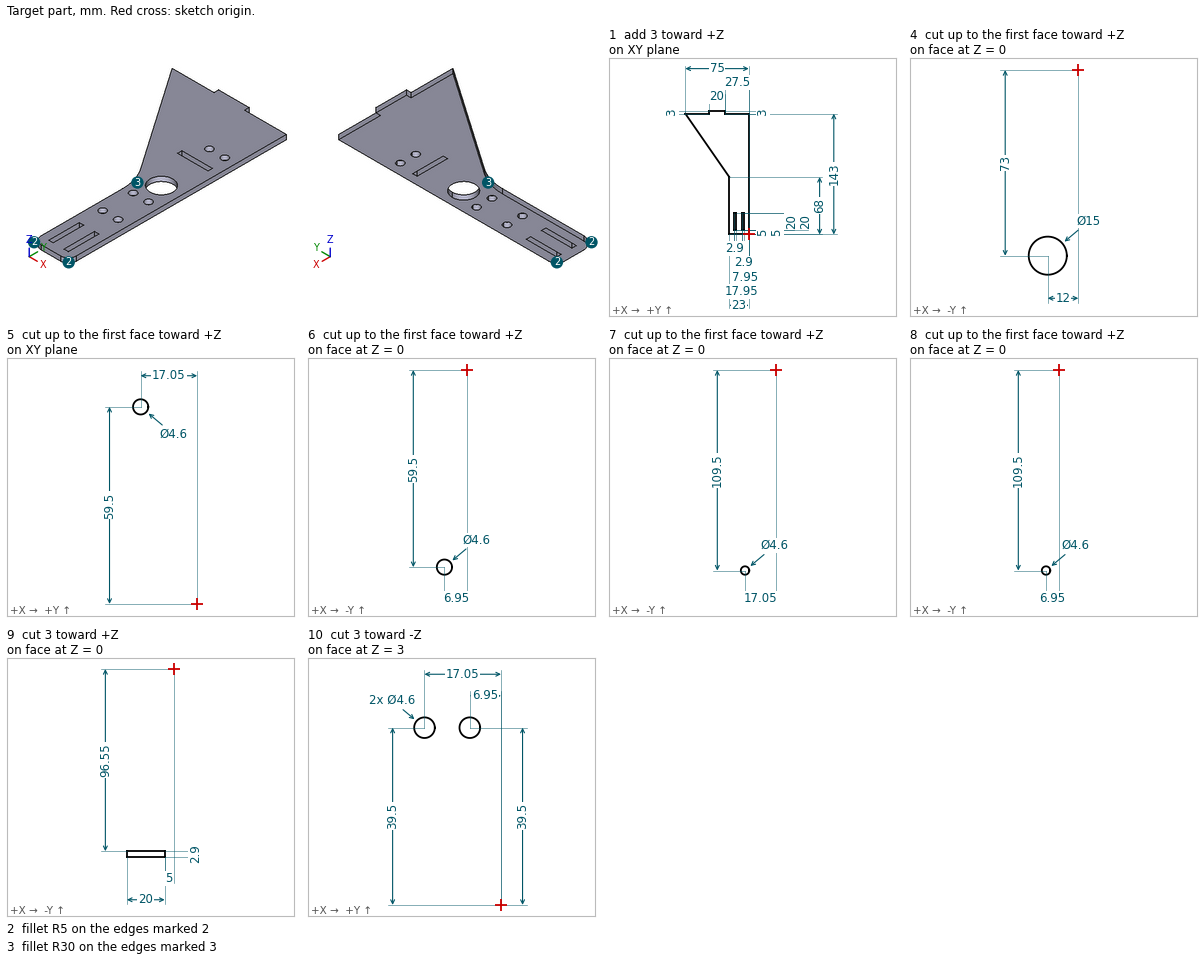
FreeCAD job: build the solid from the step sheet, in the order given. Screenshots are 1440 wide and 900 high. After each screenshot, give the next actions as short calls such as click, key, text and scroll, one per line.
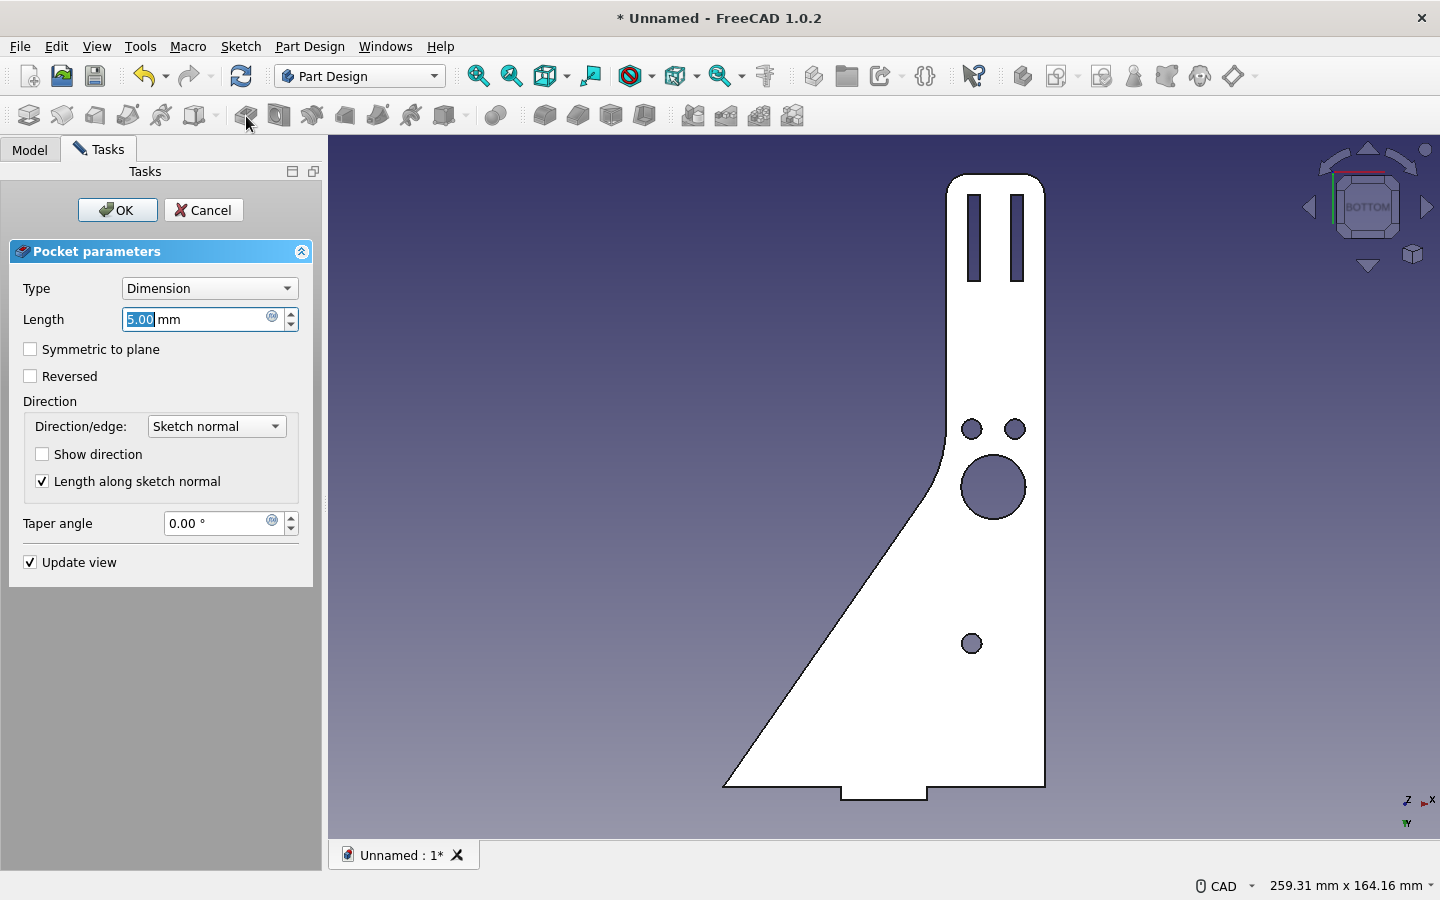
click(210, 288)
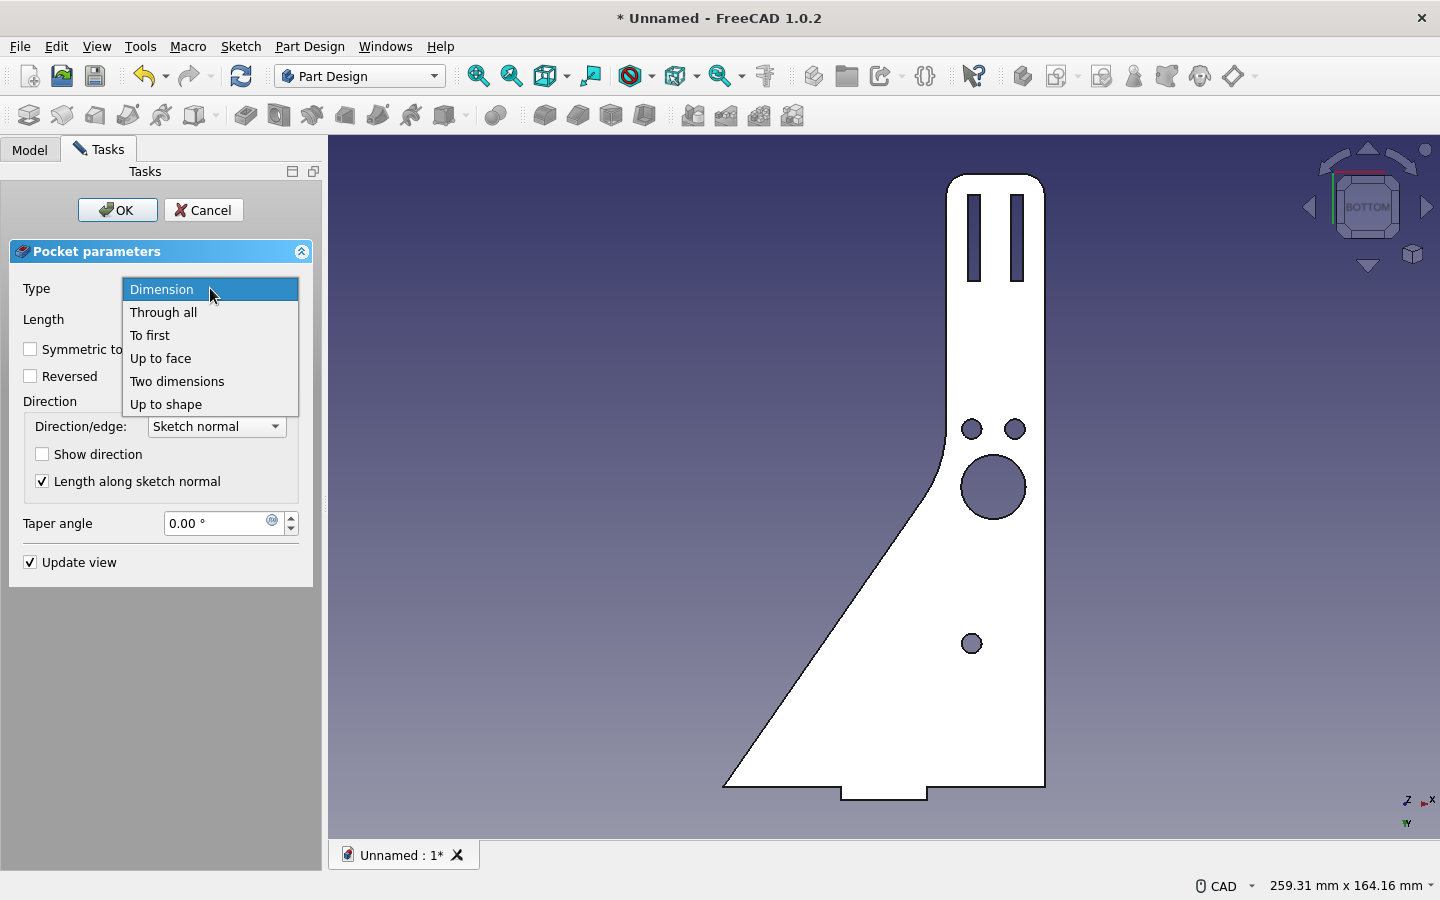
click(208, 336)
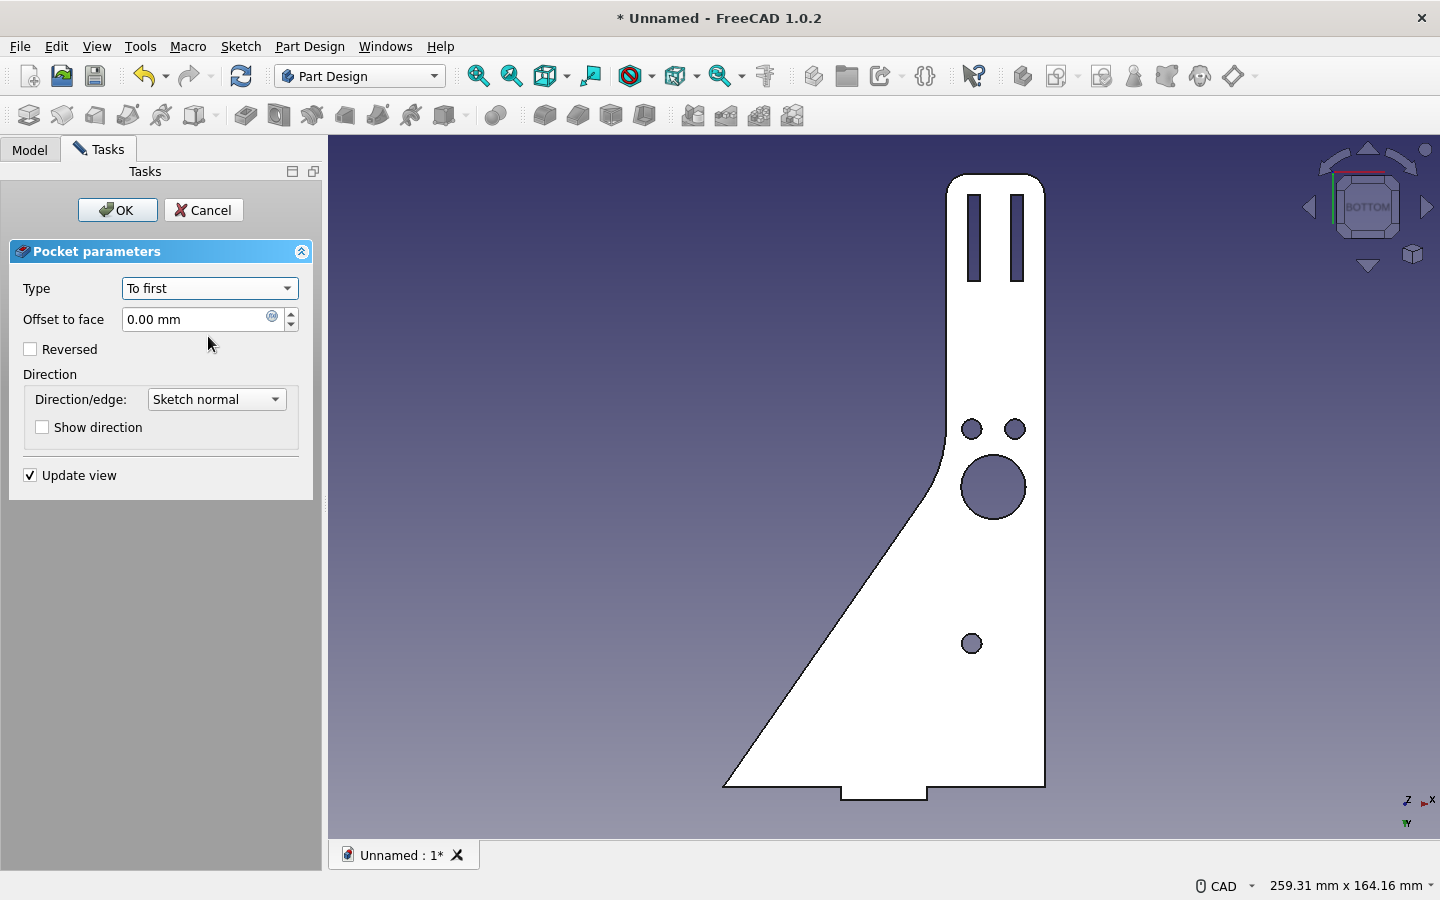
click(118, 210)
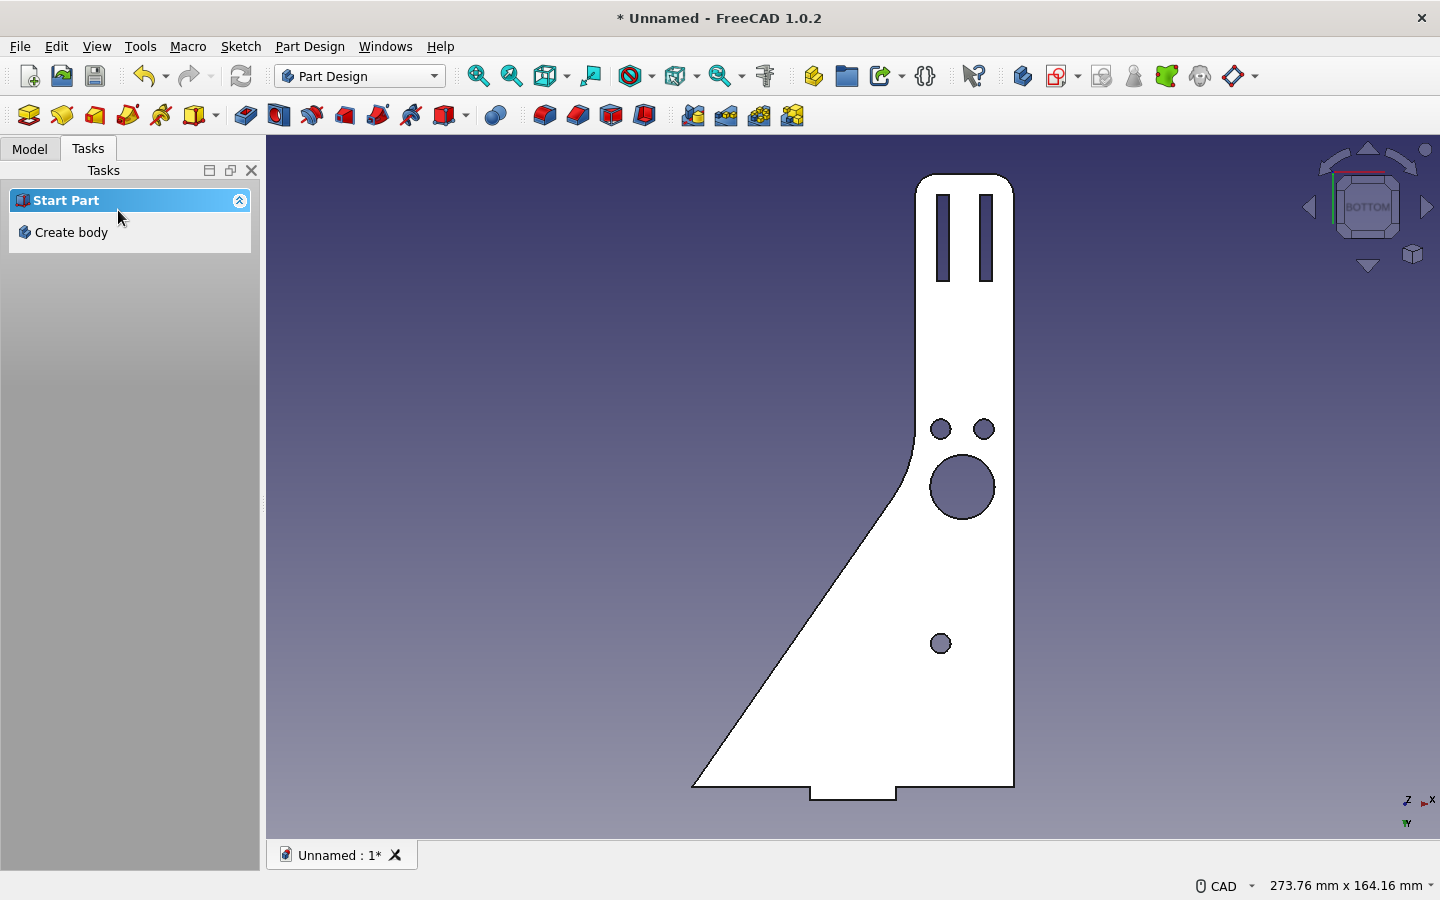
click(853, 665)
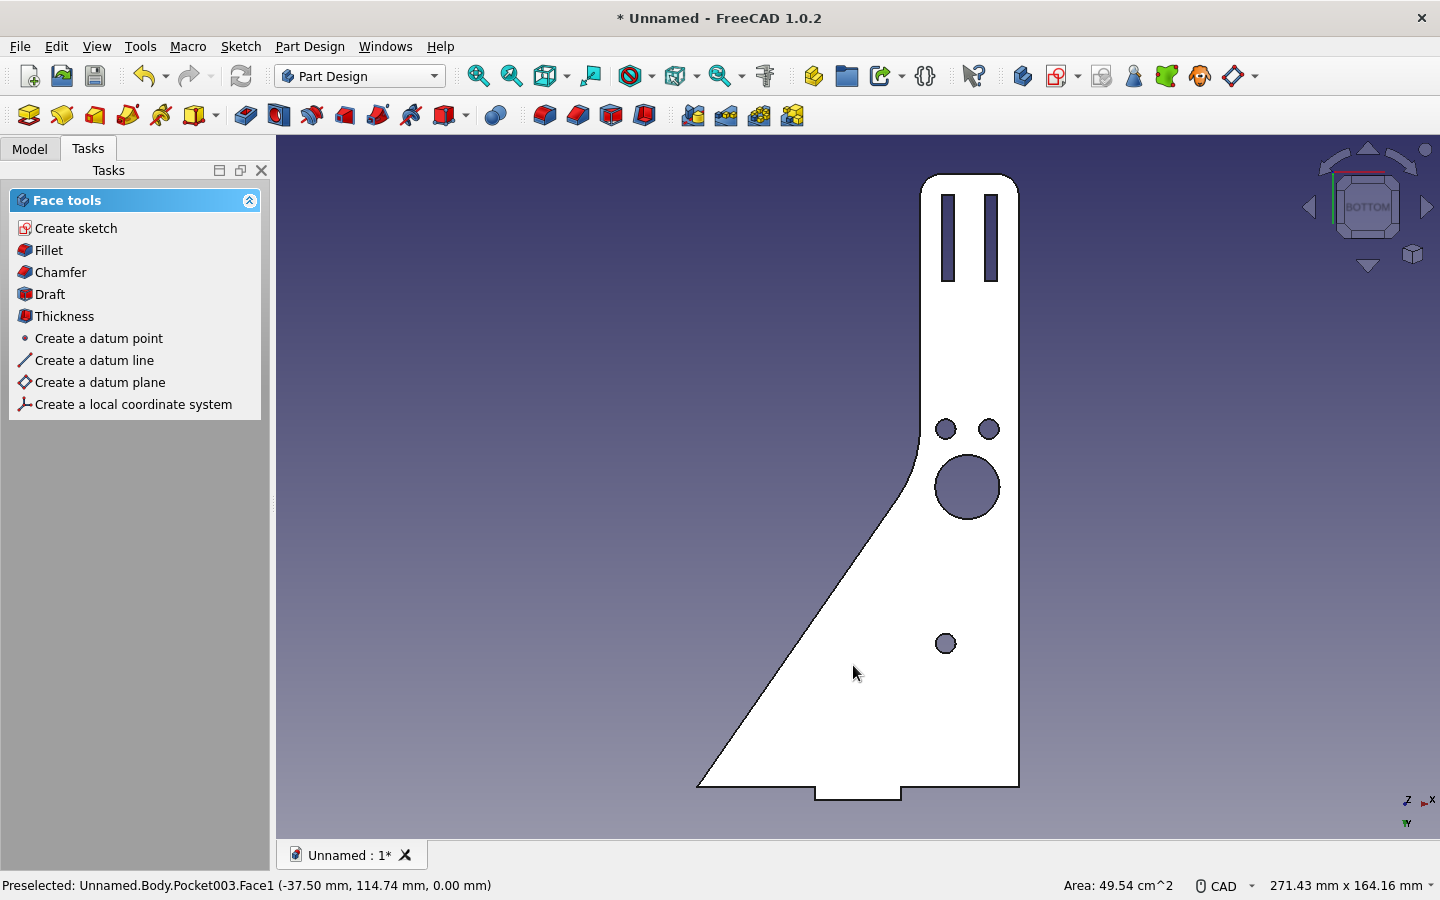
click(1056, 76)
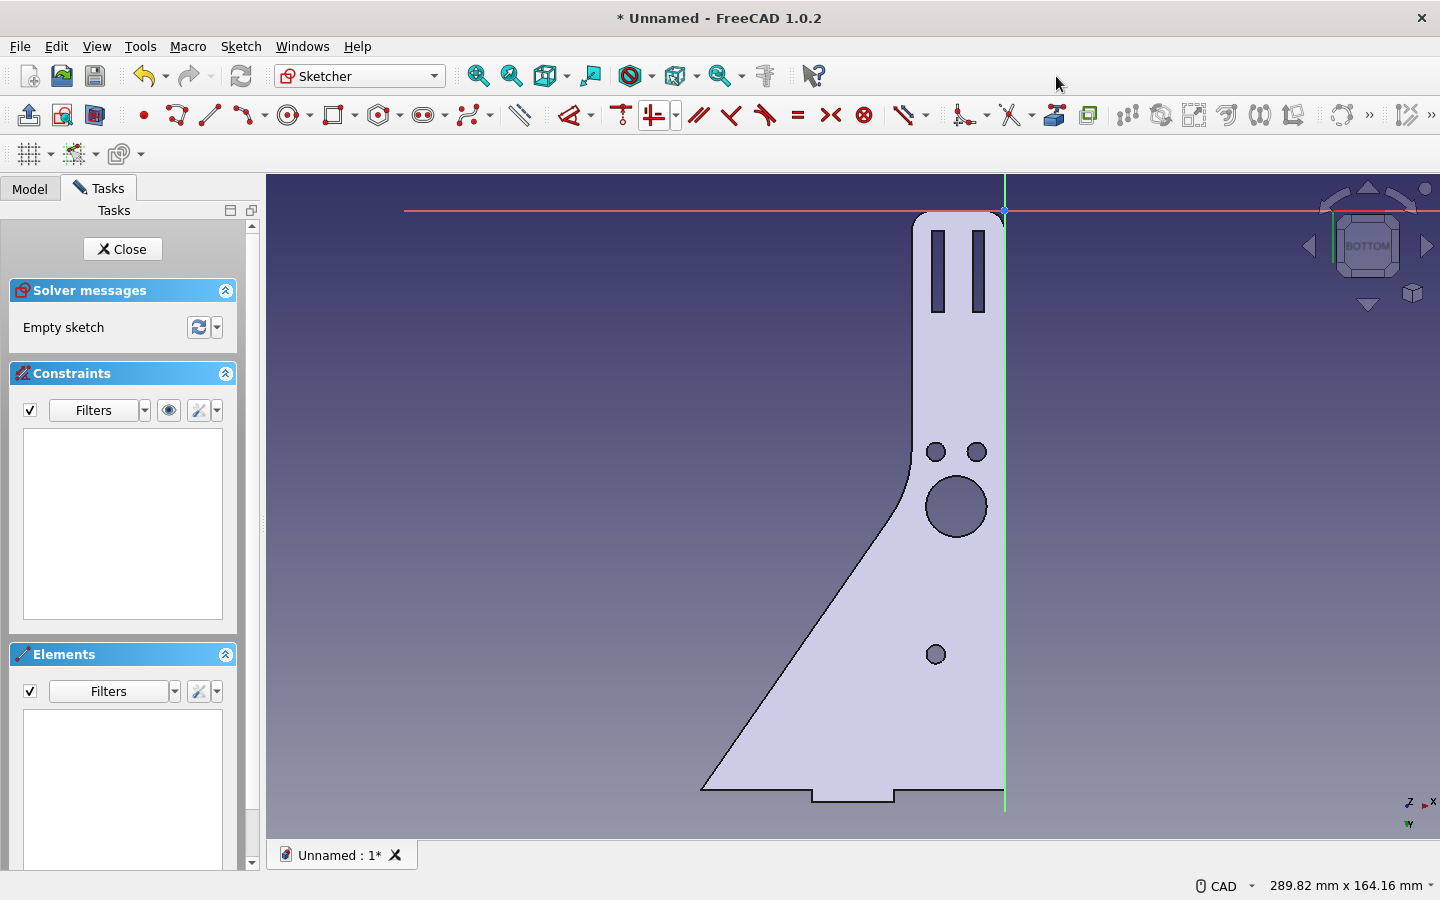
scroll(987, 662, up, 15)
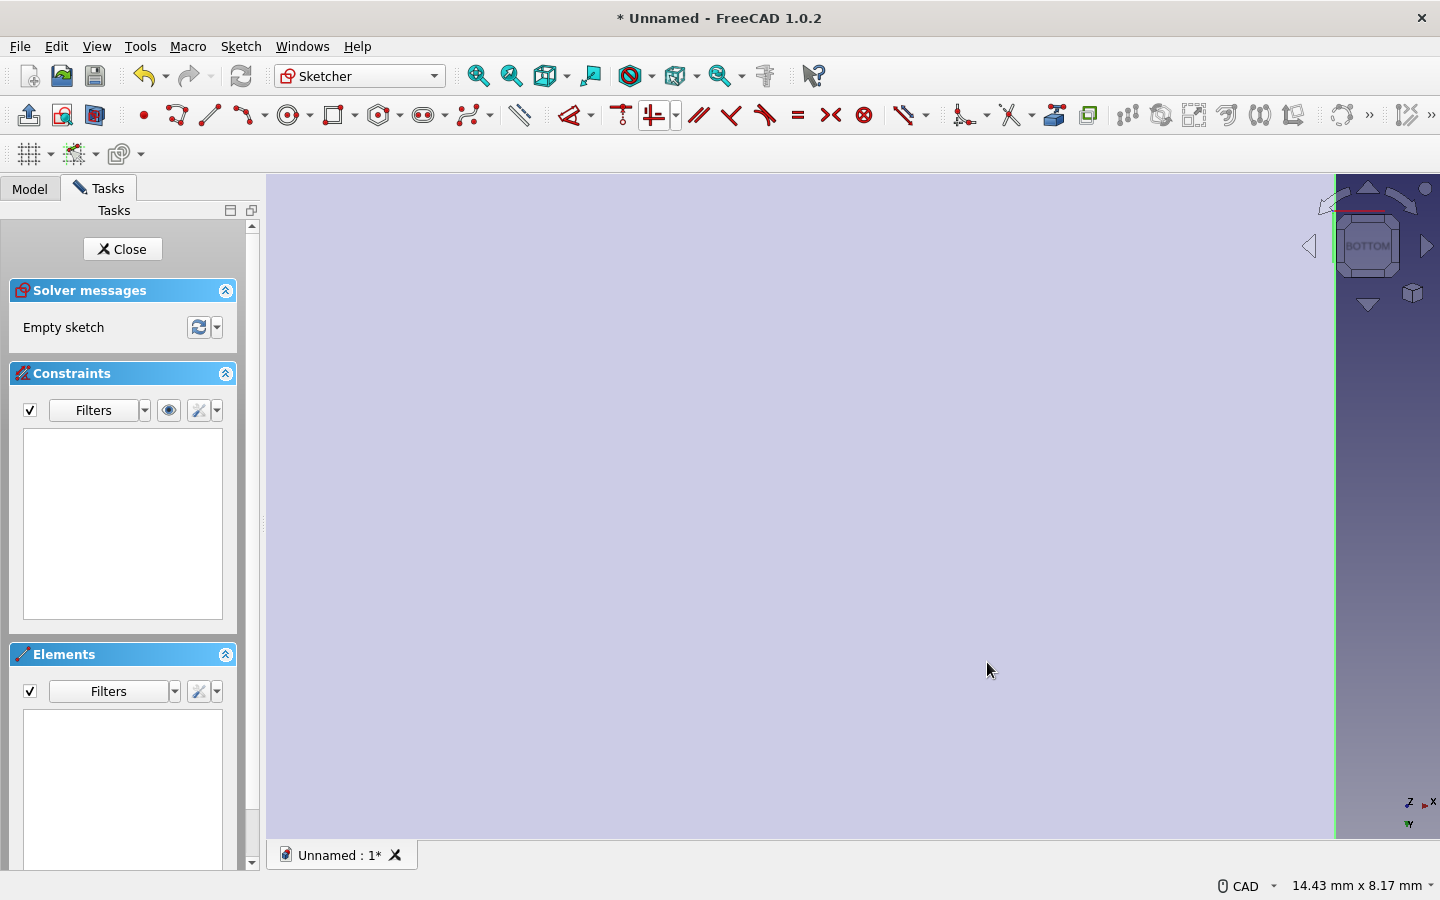
key(g)
key(c)